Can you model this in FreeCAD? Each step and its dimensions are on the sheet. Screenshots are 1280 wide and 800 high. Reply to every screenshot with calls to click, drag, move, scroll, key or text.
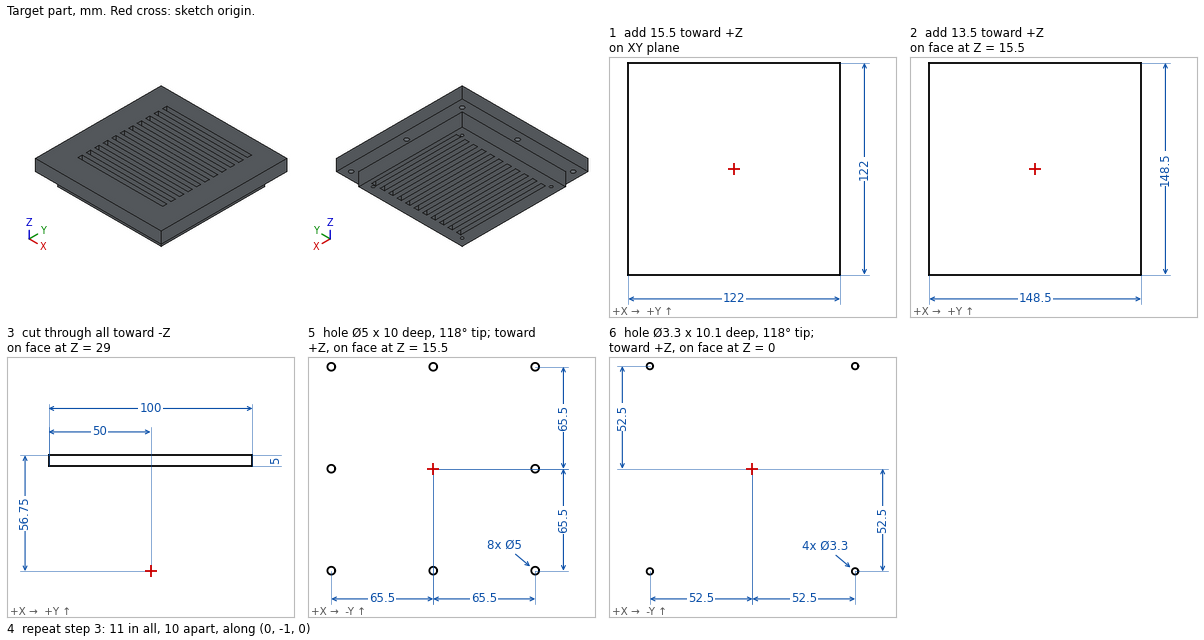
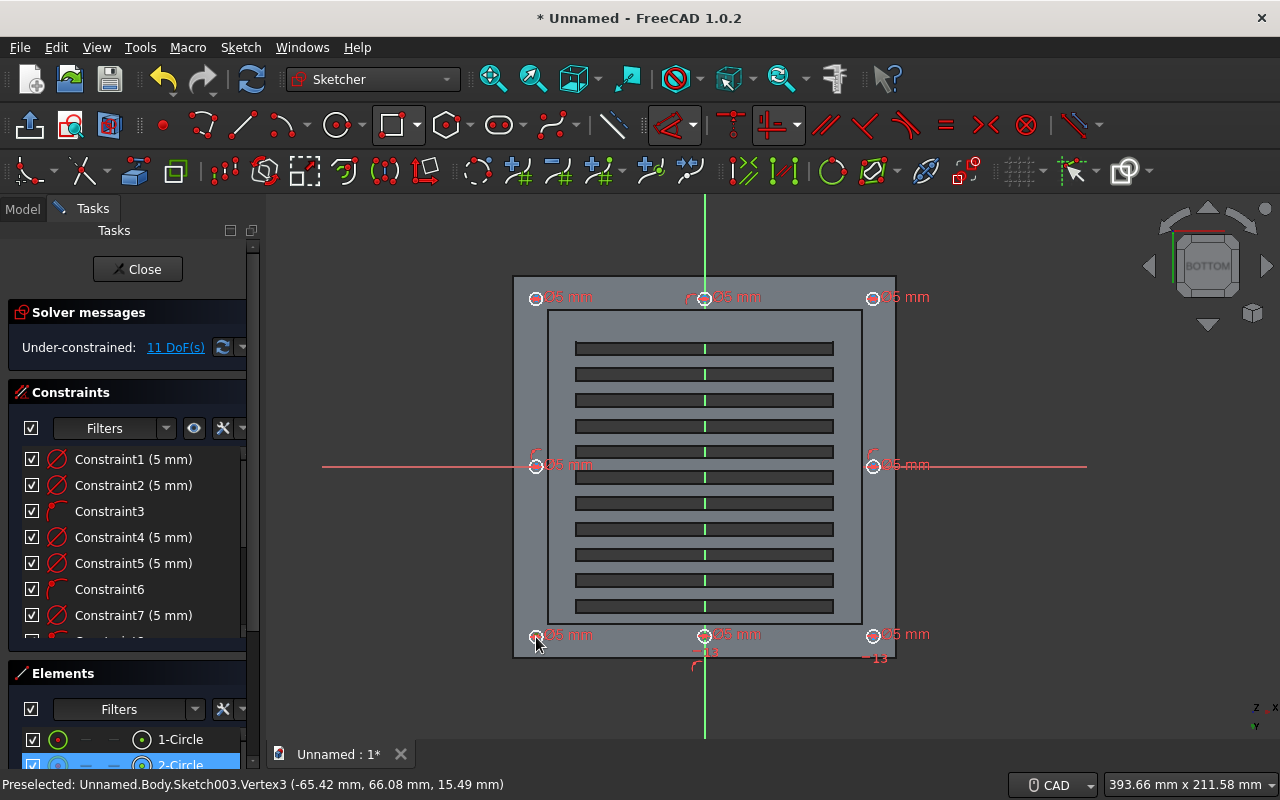
key(h)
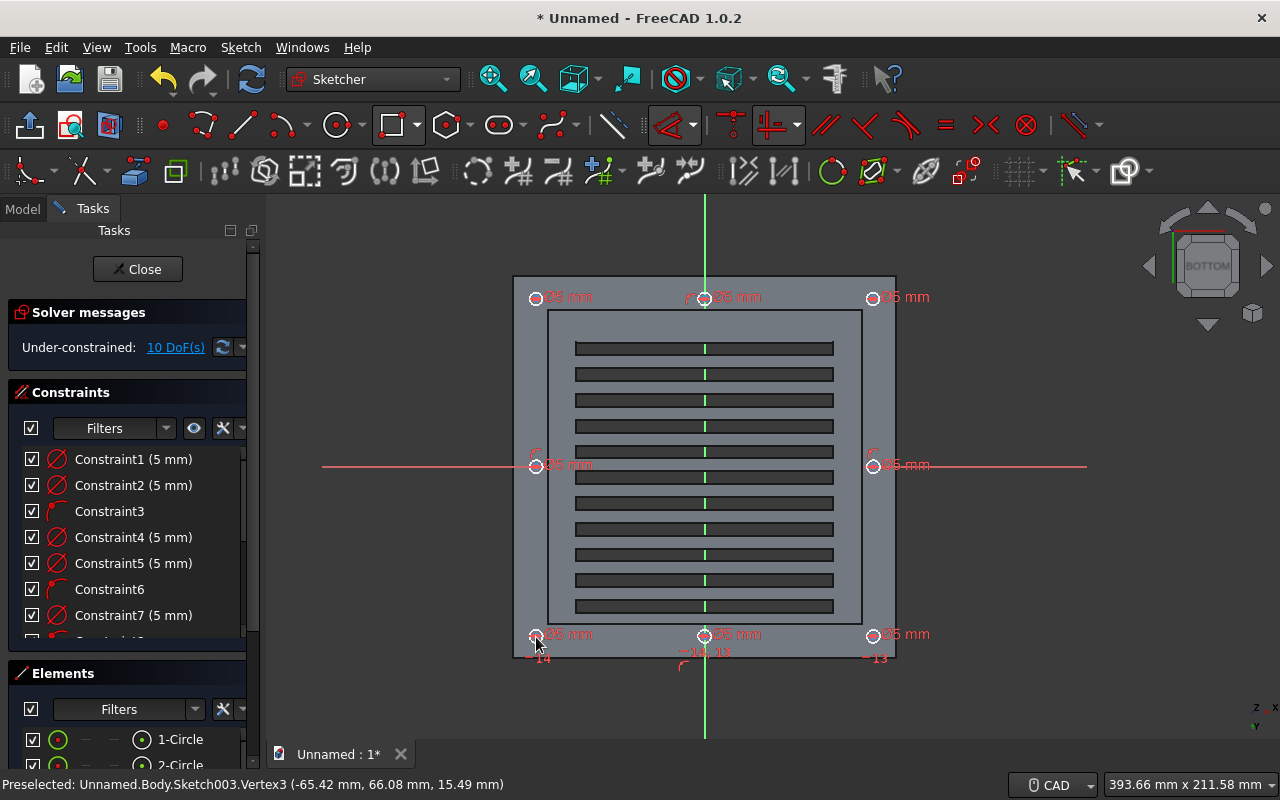
click(536, 636)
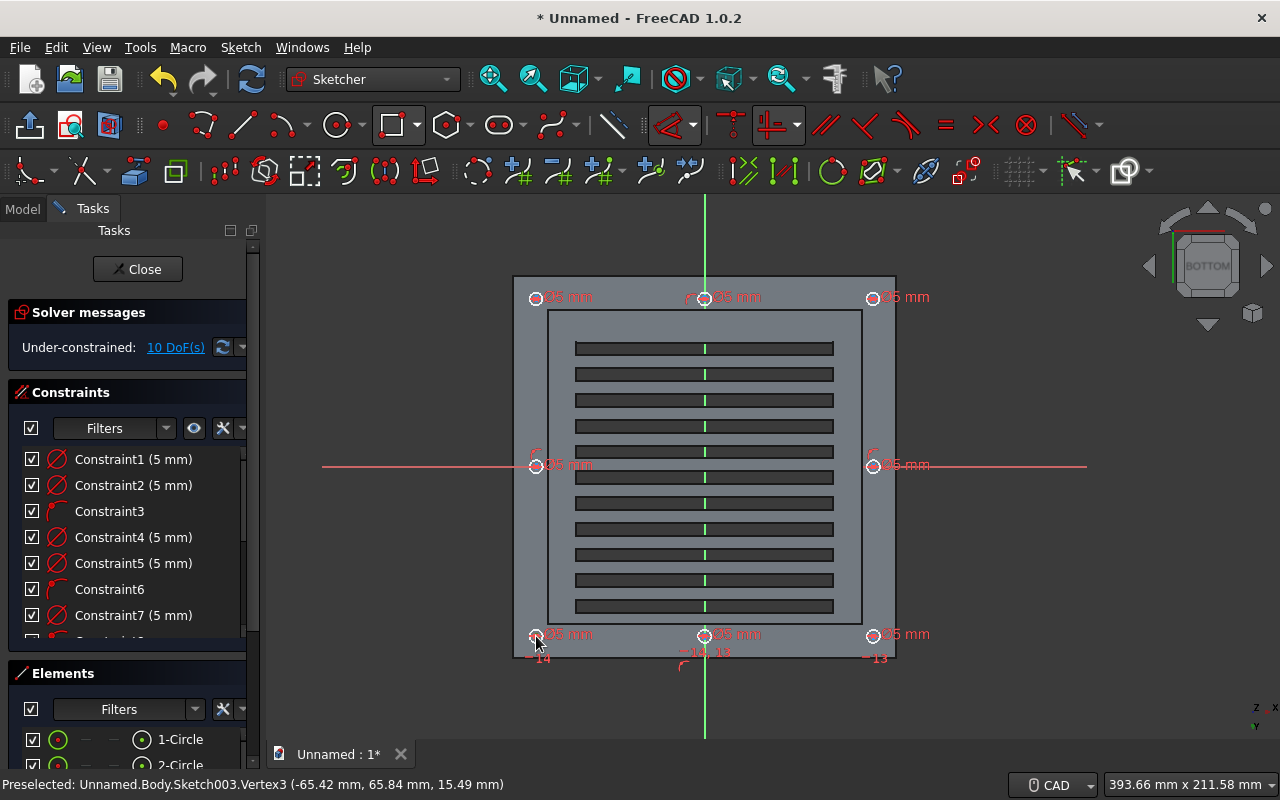
click(536, 467)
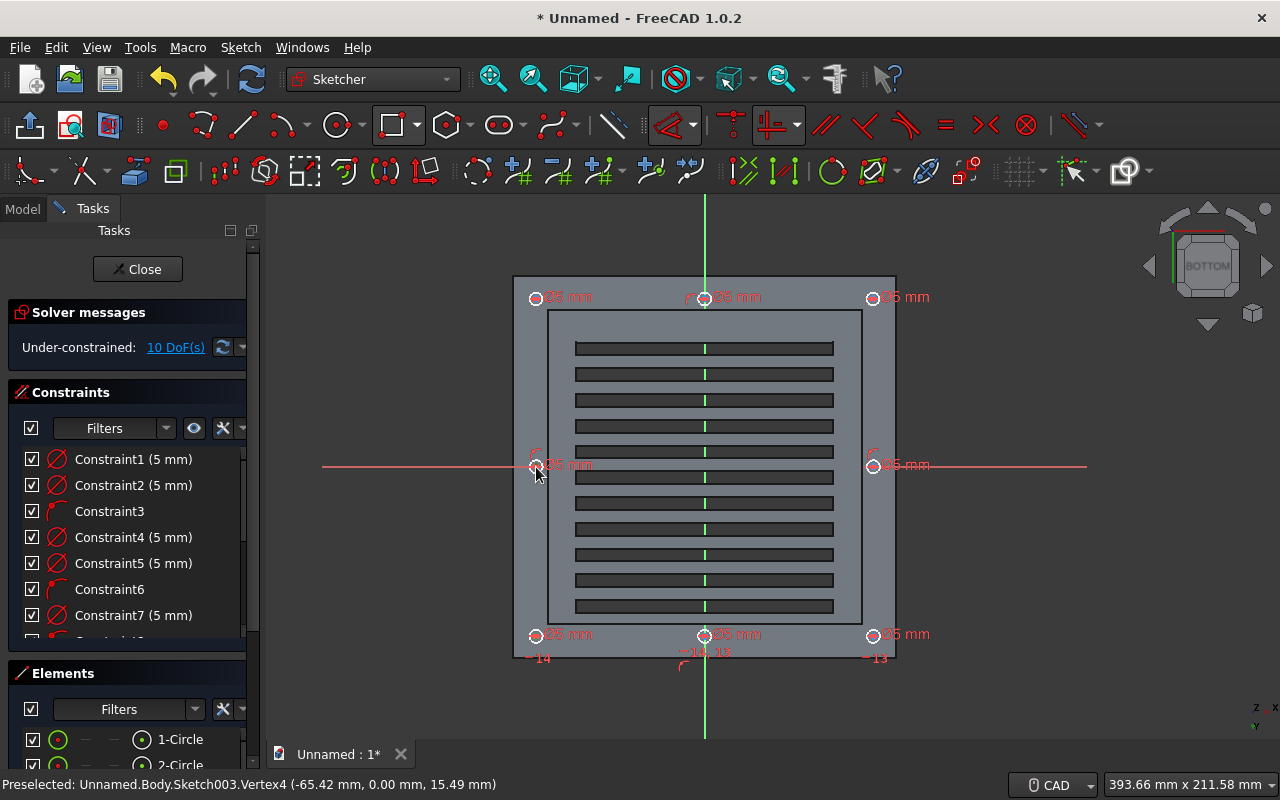
click(800, 126)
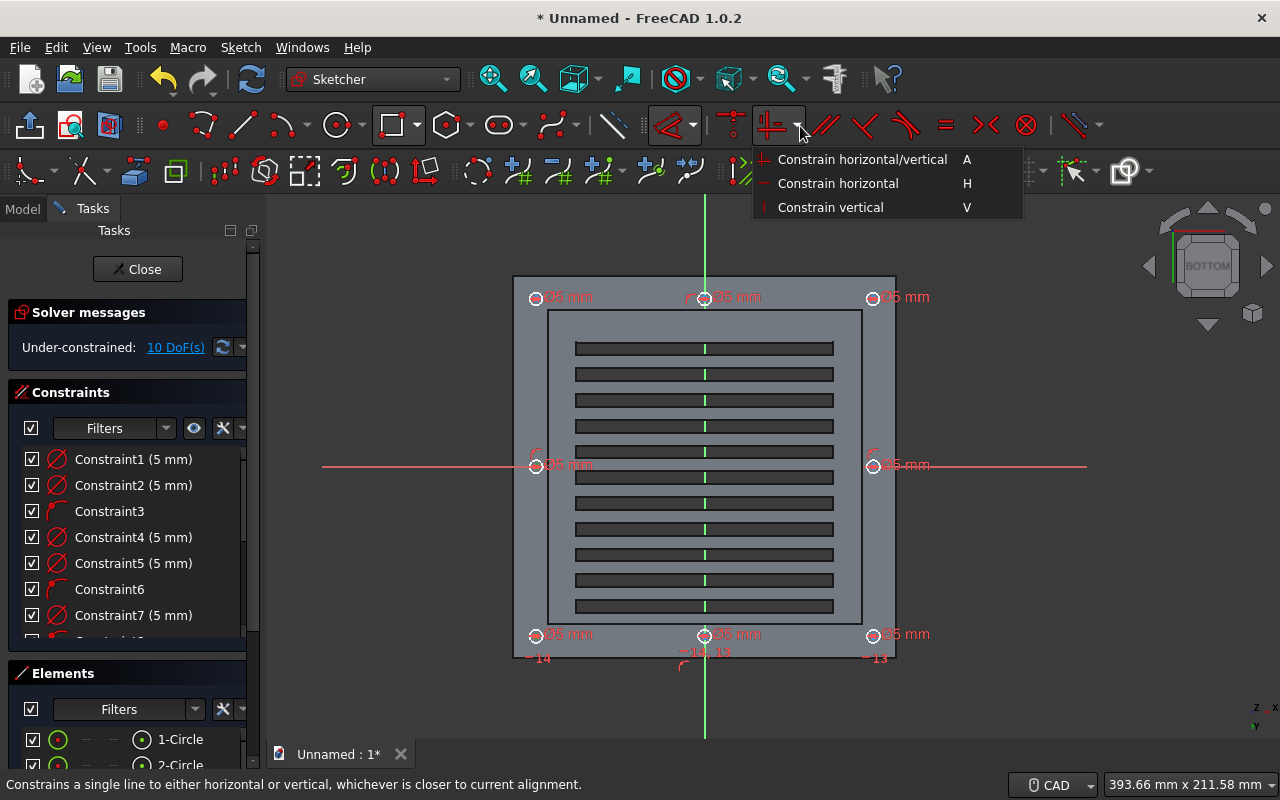
click(888, 207)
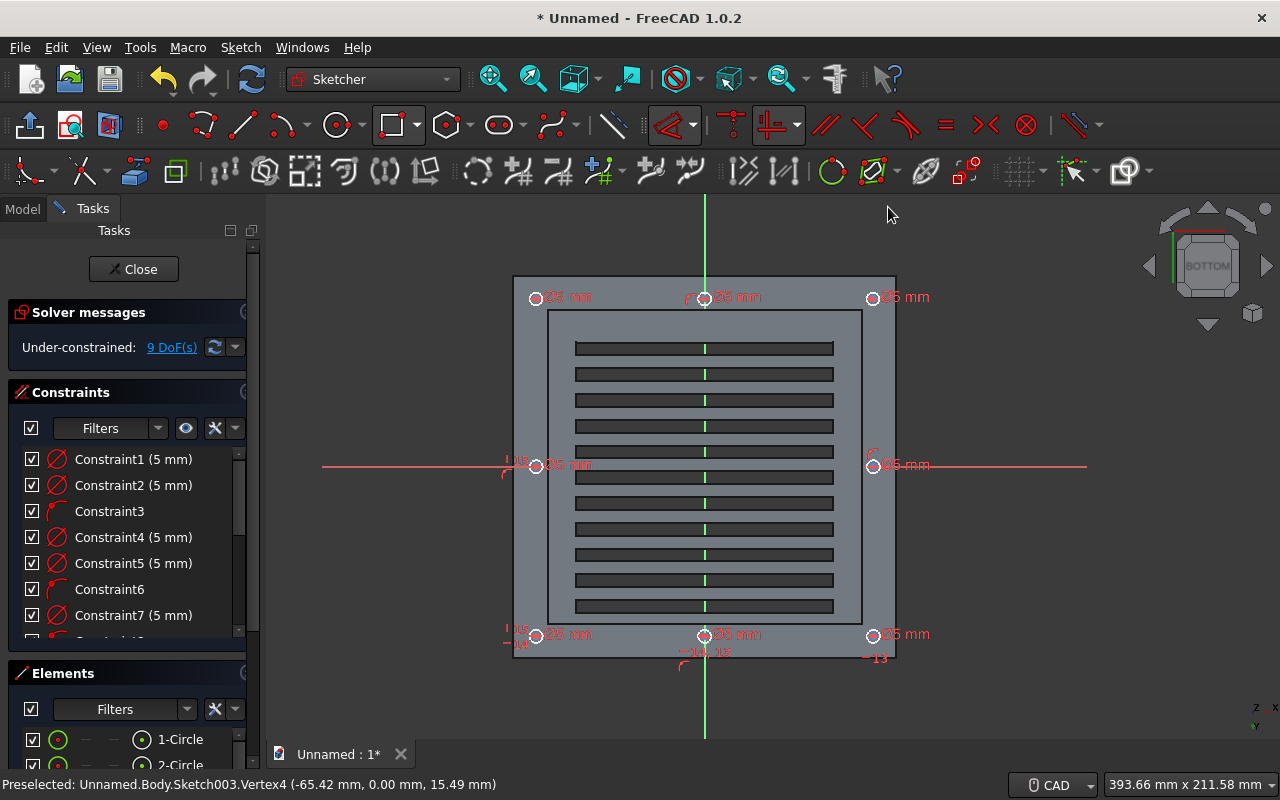
click(873, 636)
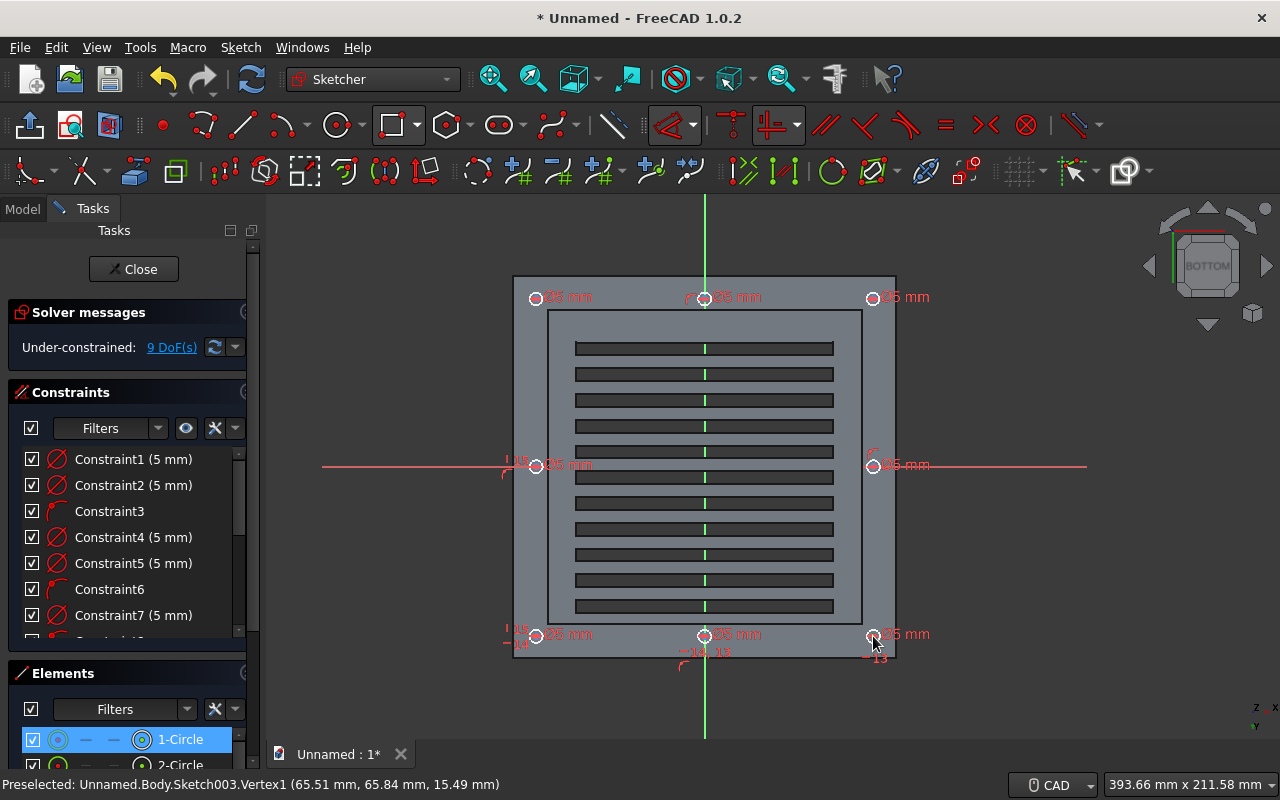
click(873, 467)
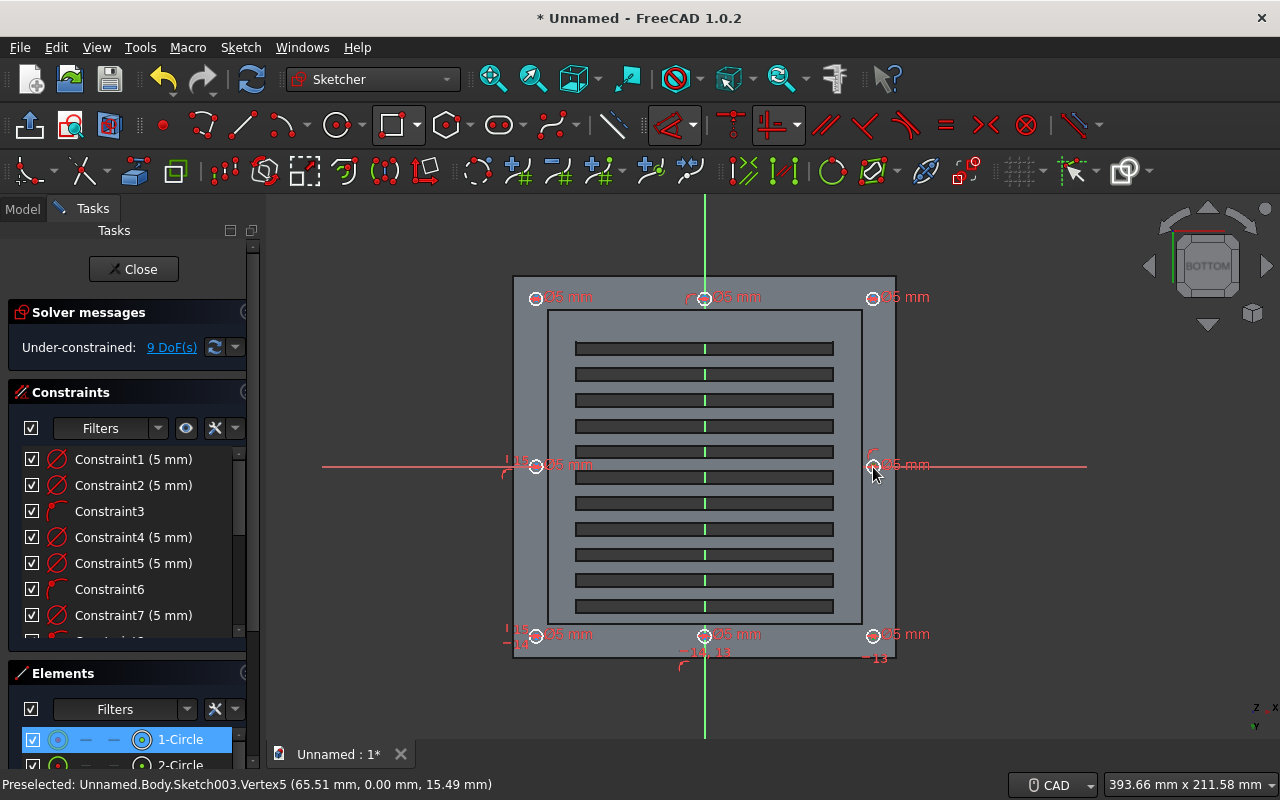
click(800, 126)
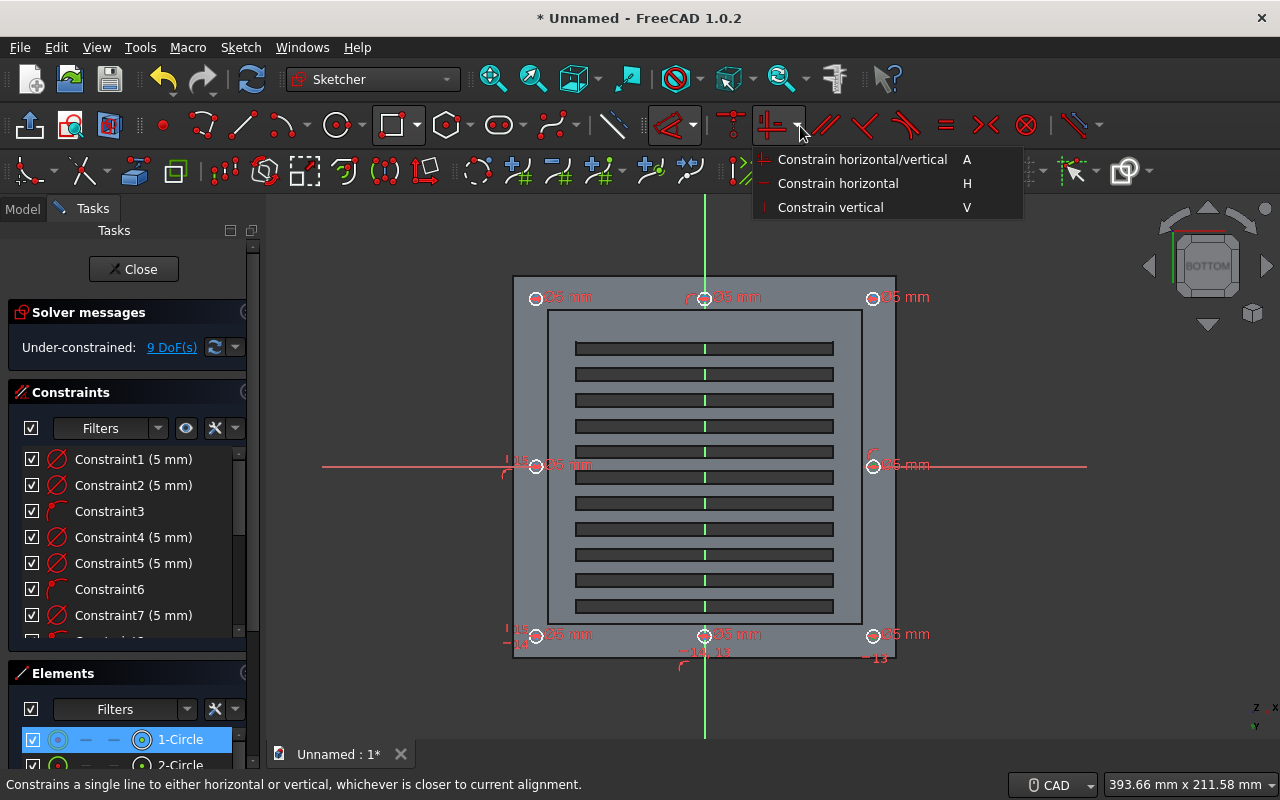
click(888, 207)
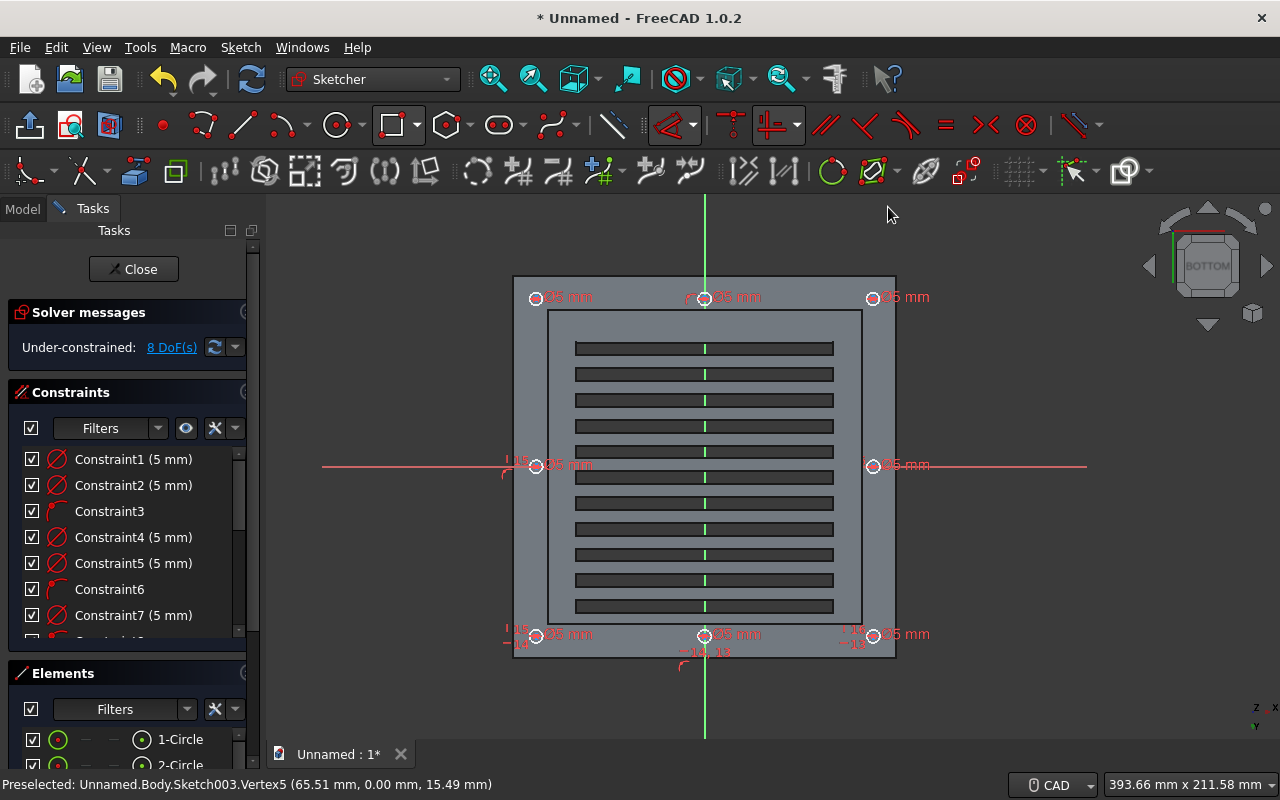
click(873, 467)